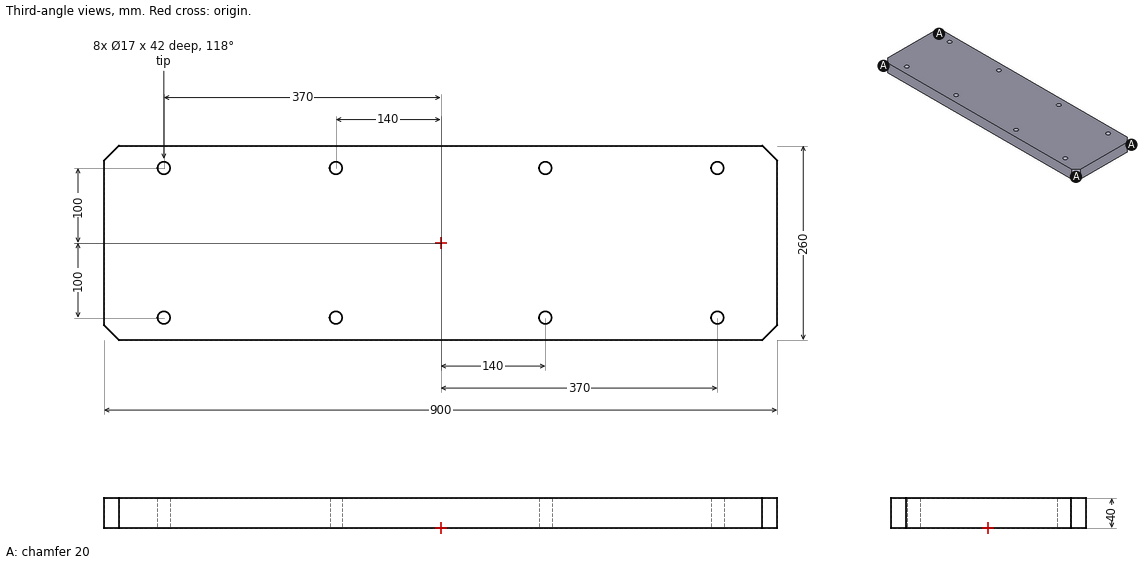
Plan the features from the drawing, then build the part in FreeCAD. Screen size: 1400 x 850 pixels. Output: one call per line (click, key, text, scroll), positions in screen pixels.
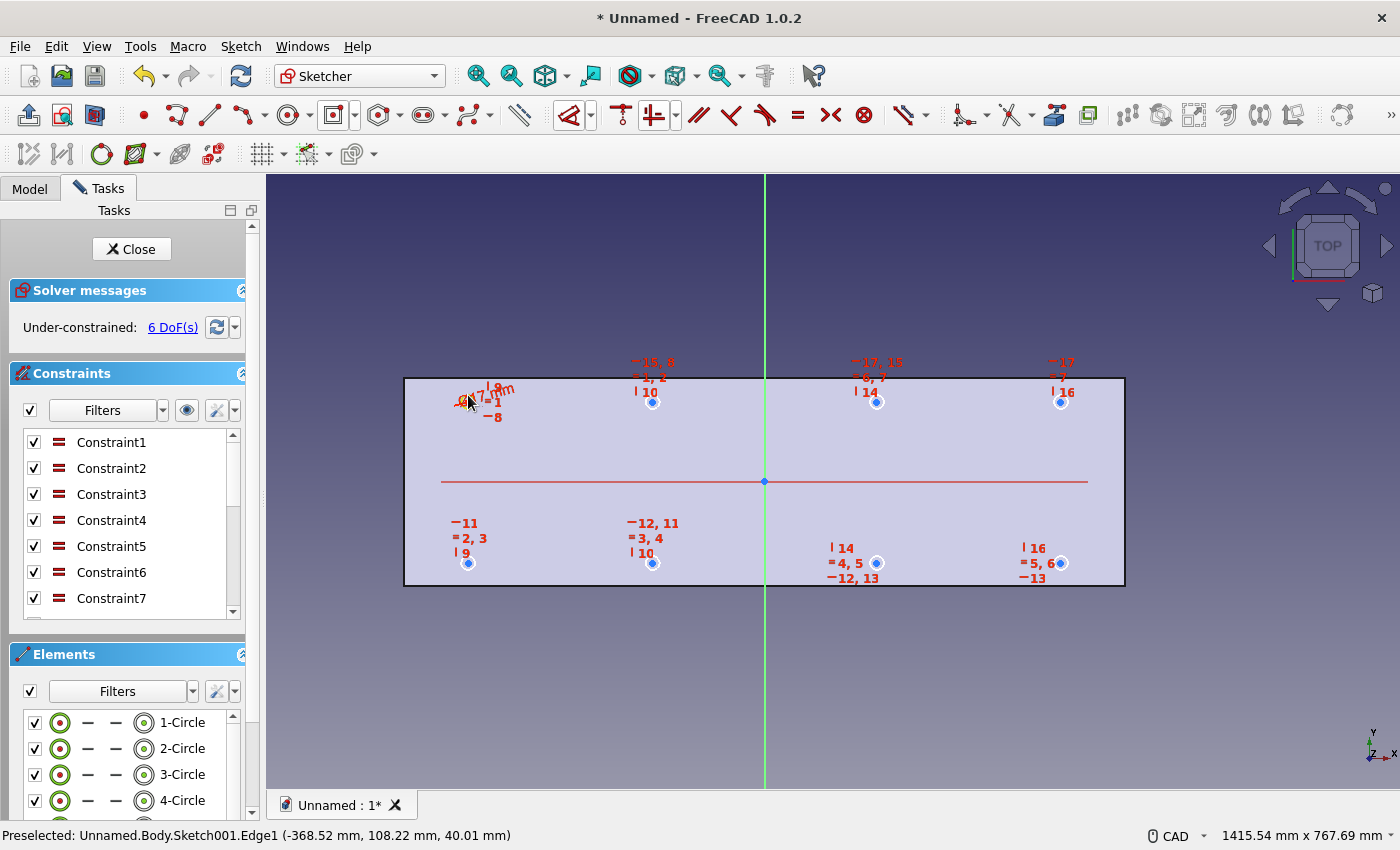
click(468, 402)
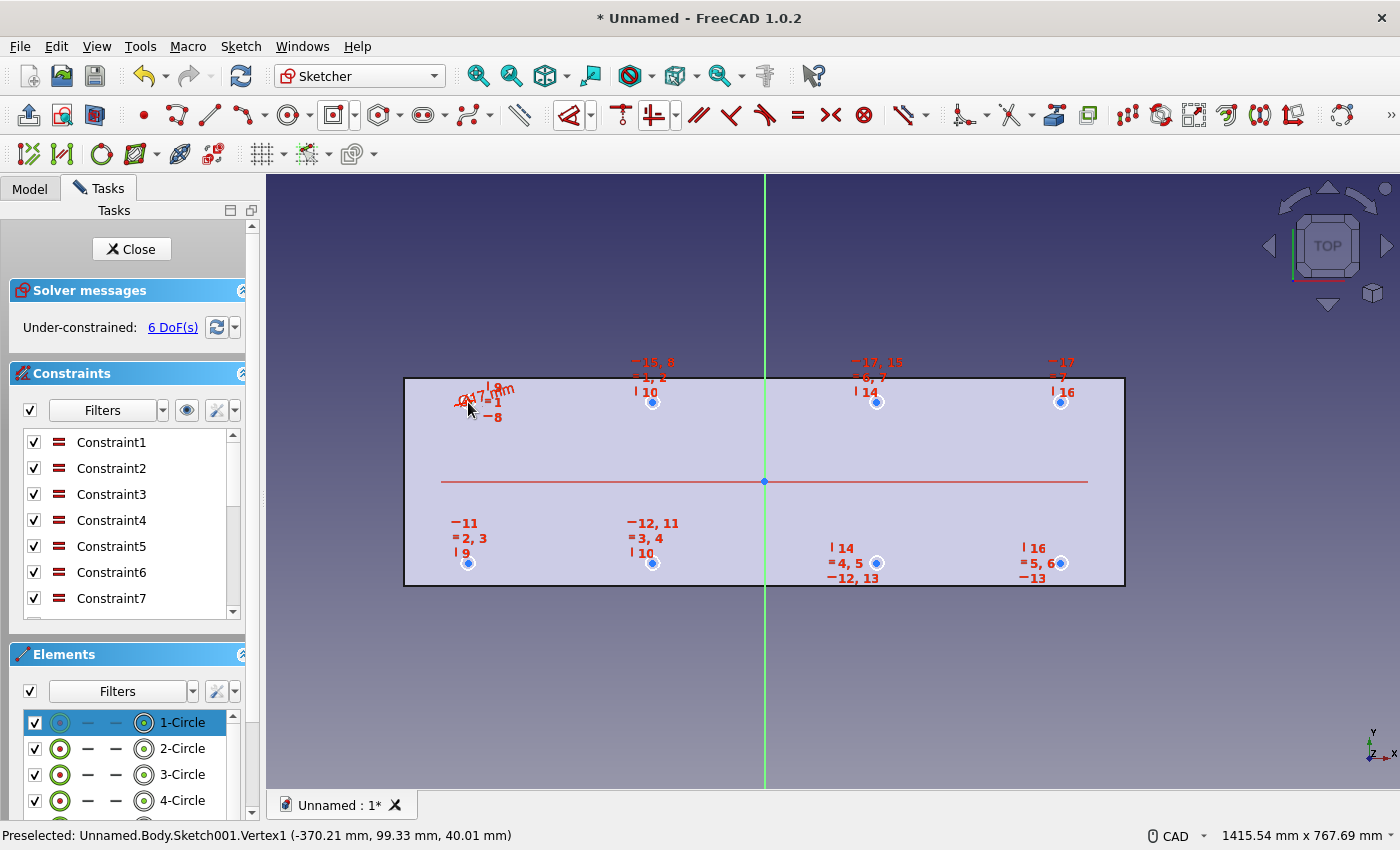
key(l)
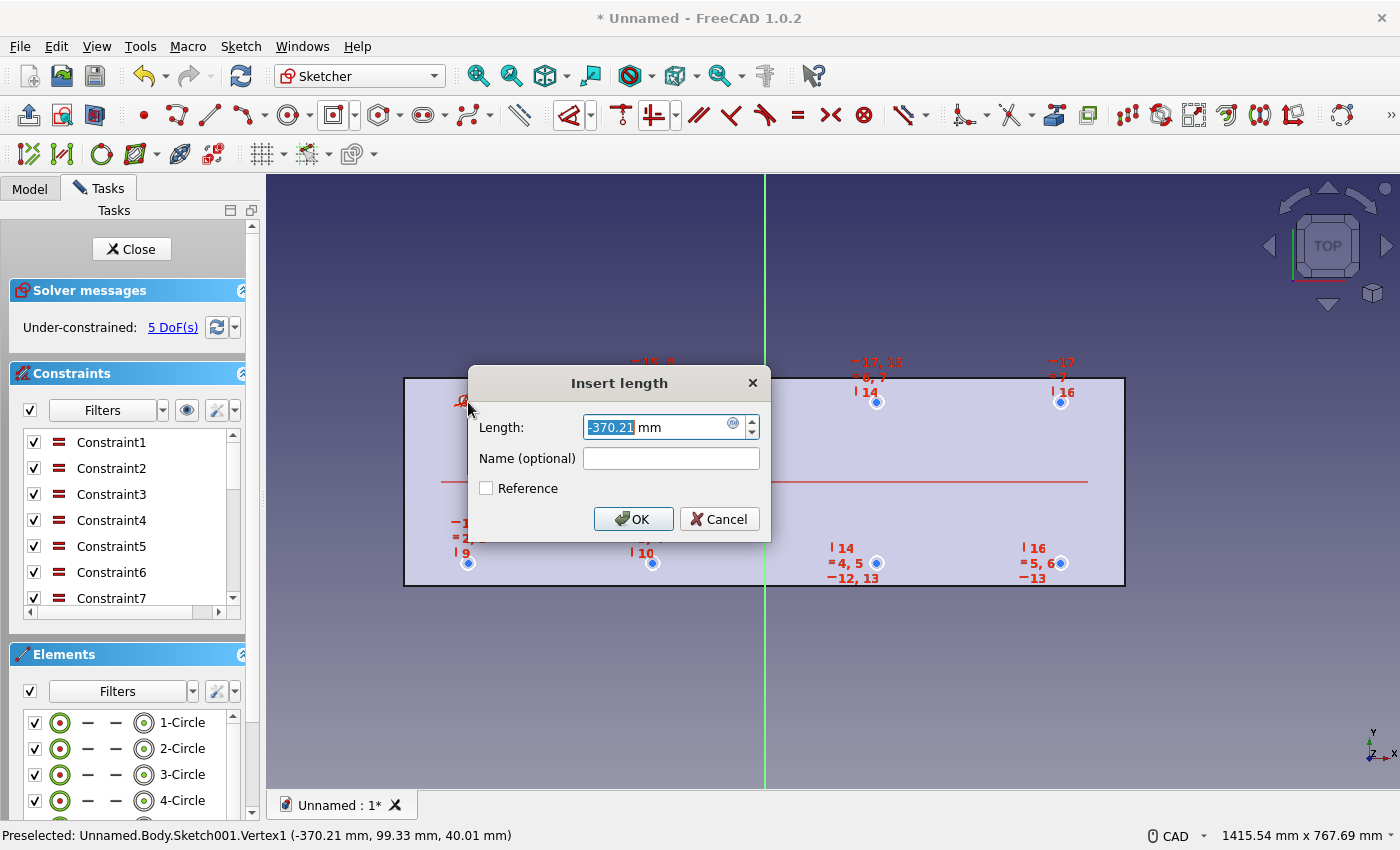
text(-370)
key(Return)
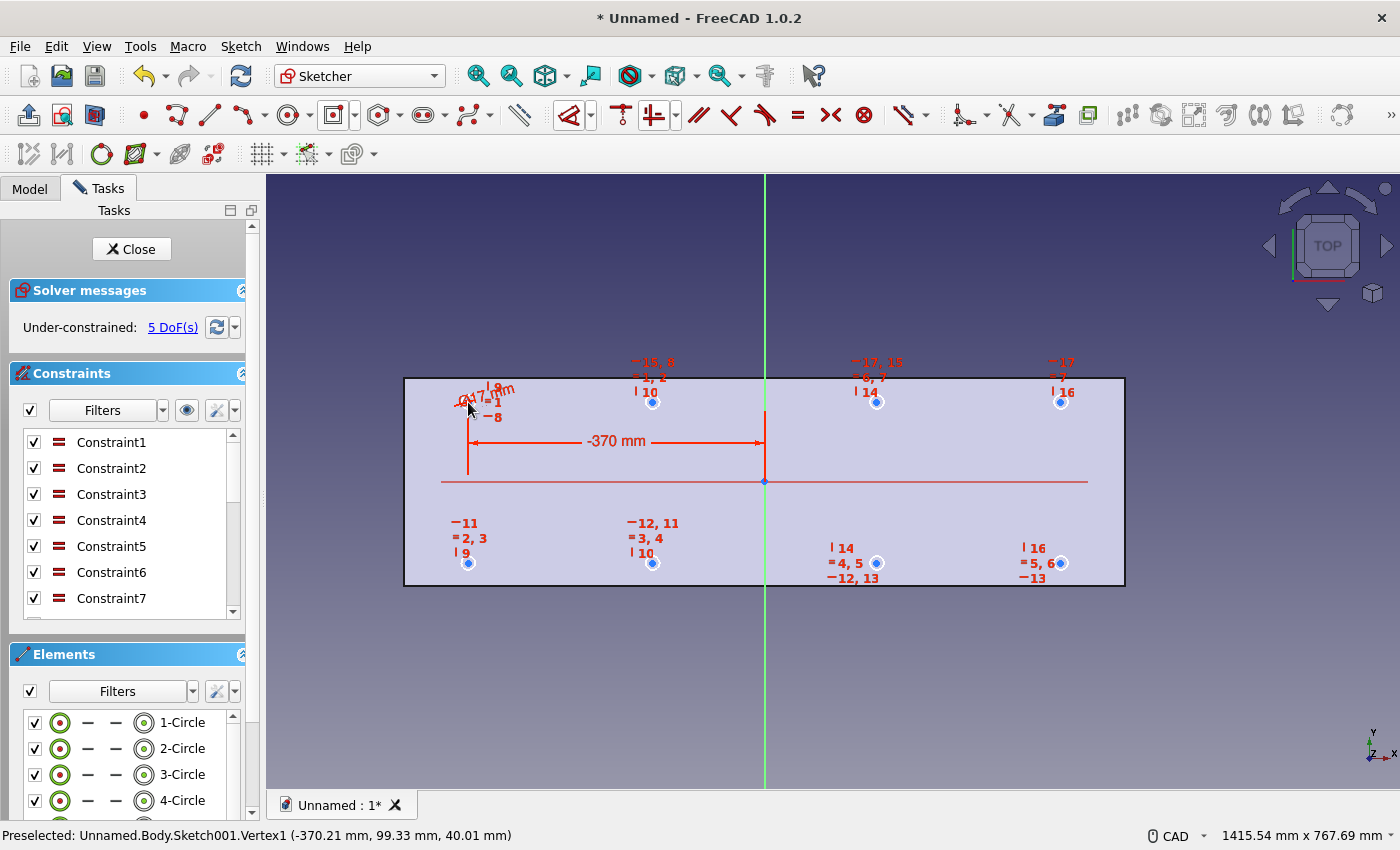
click(468, 402)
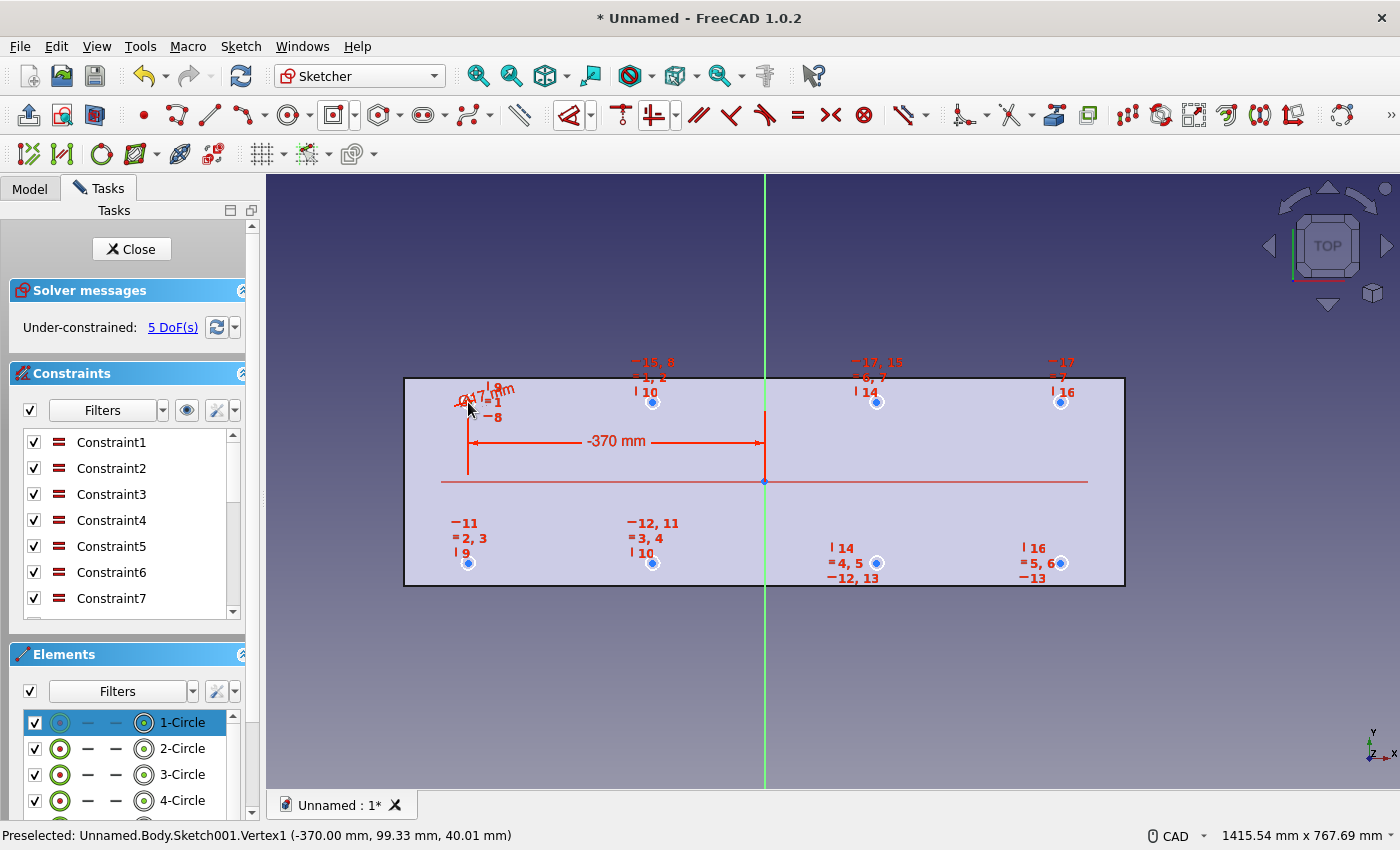
click(590, 116)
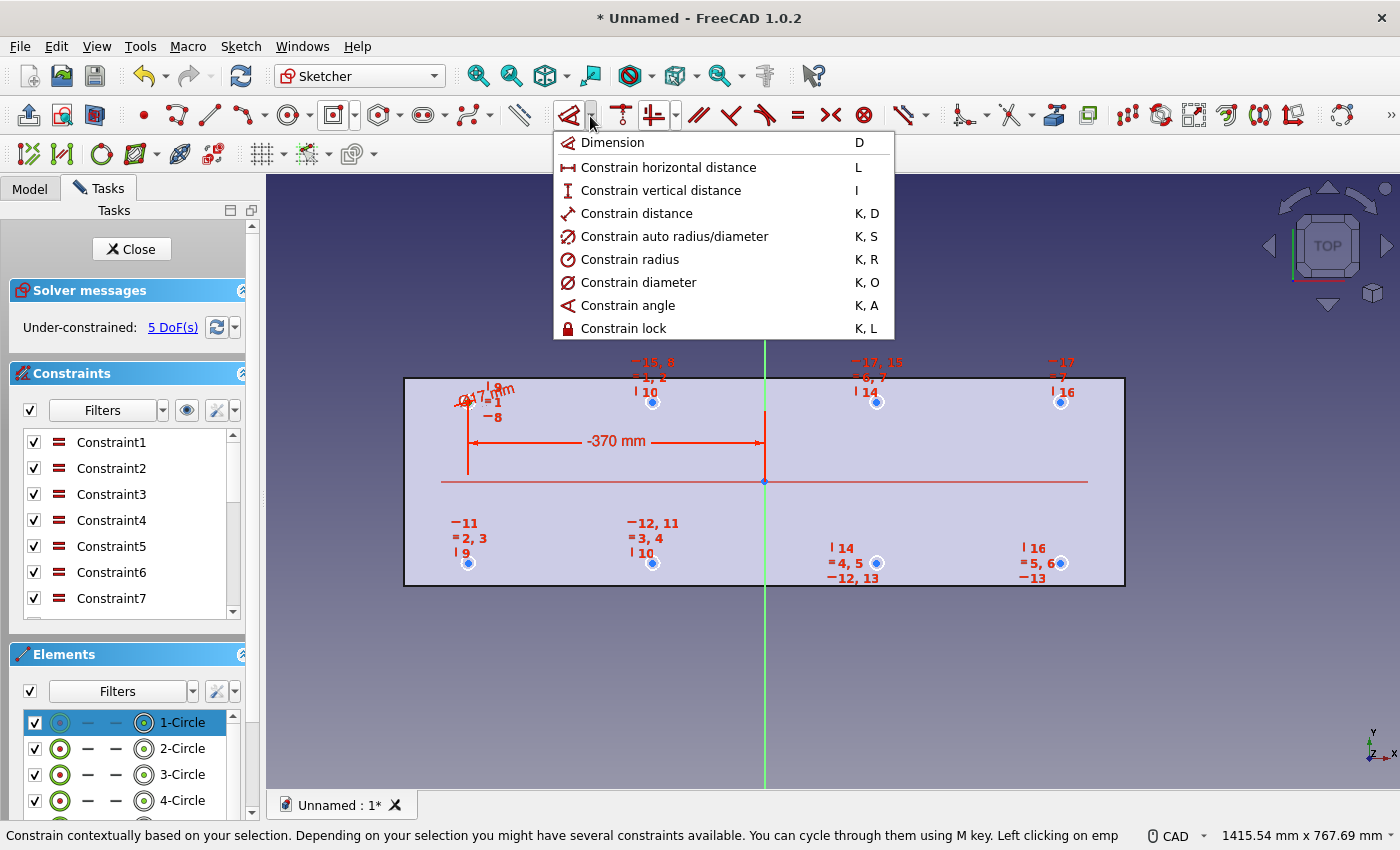
click(724, 190)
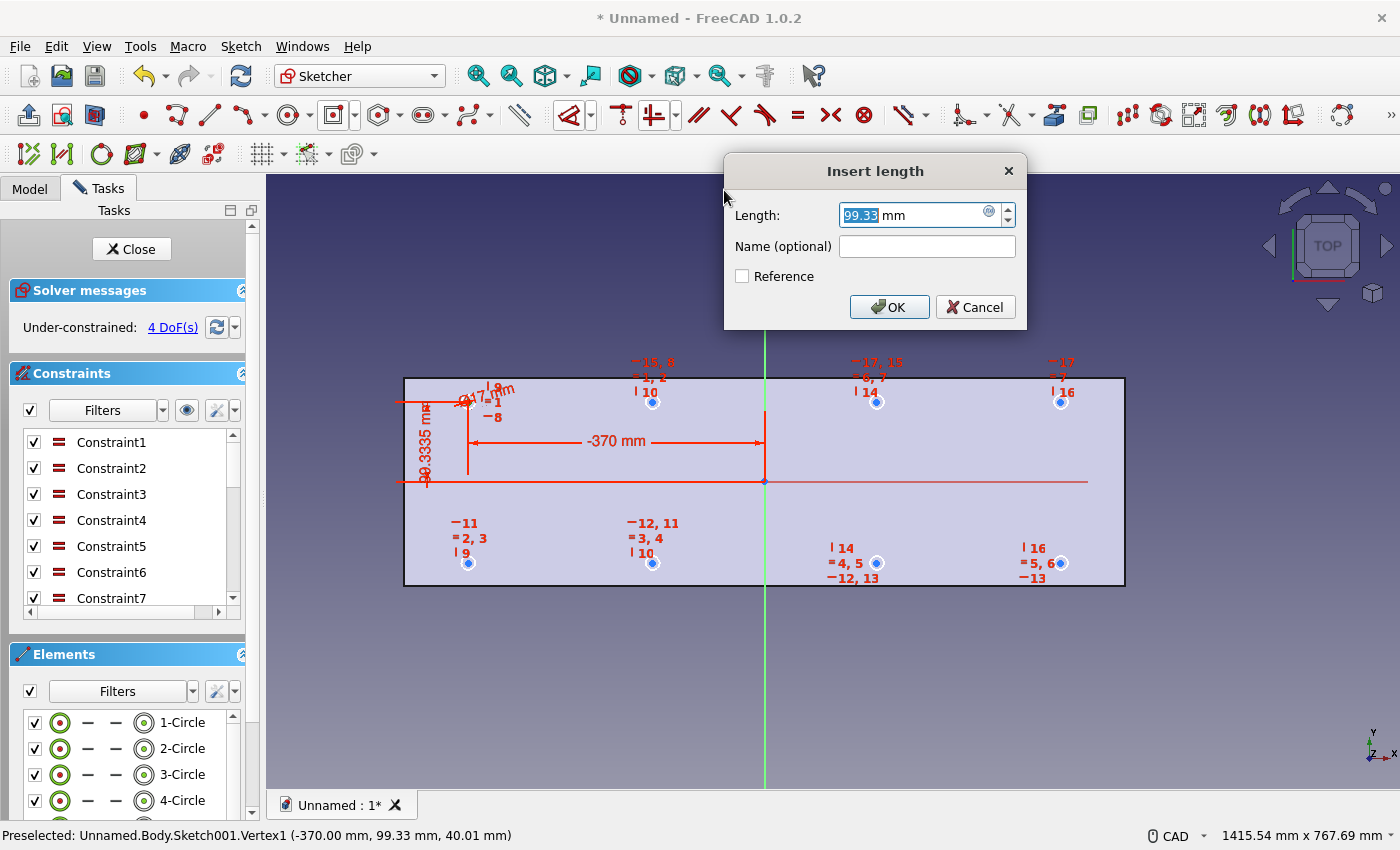
text(100)
key(Return)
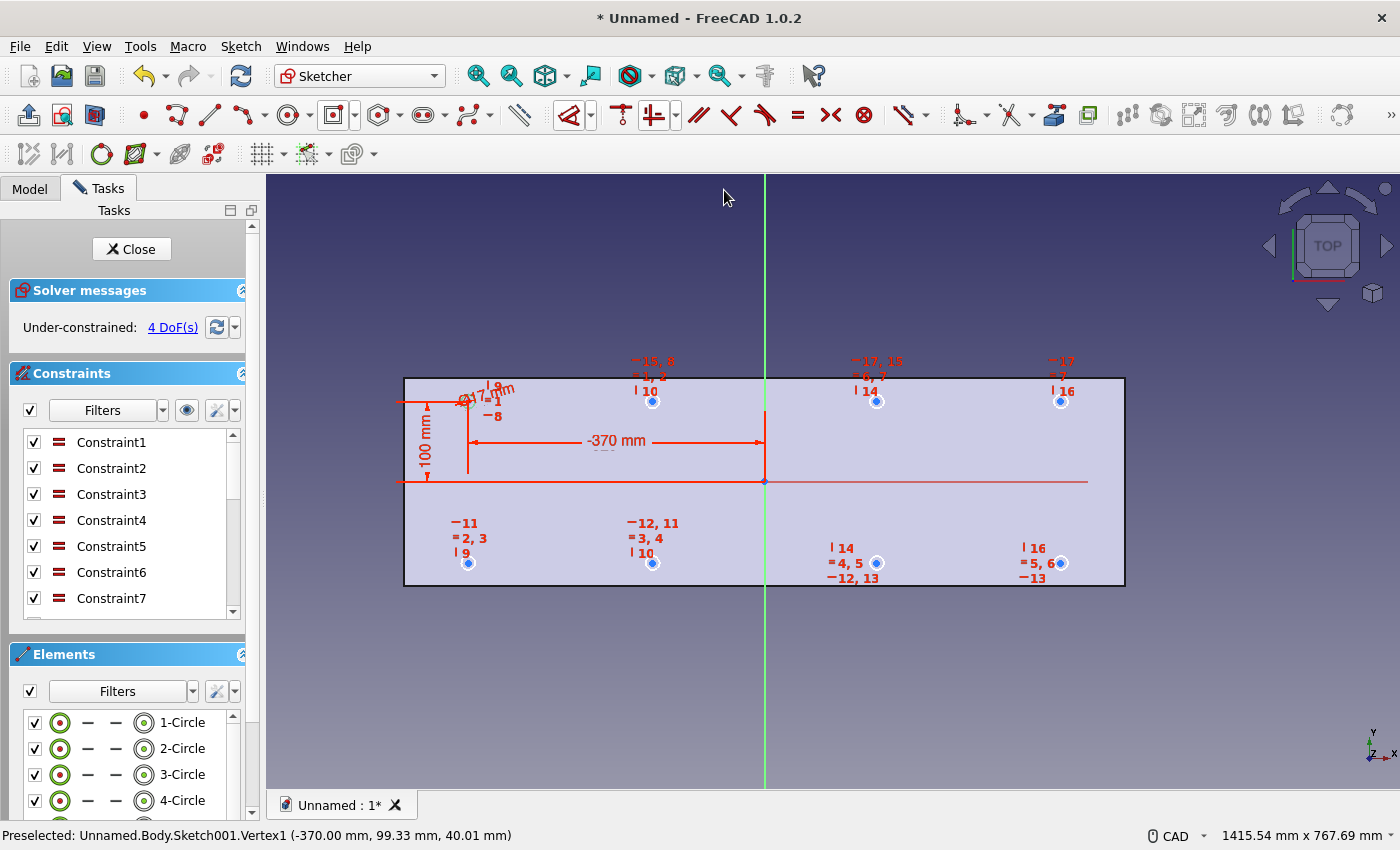
click(653, 402)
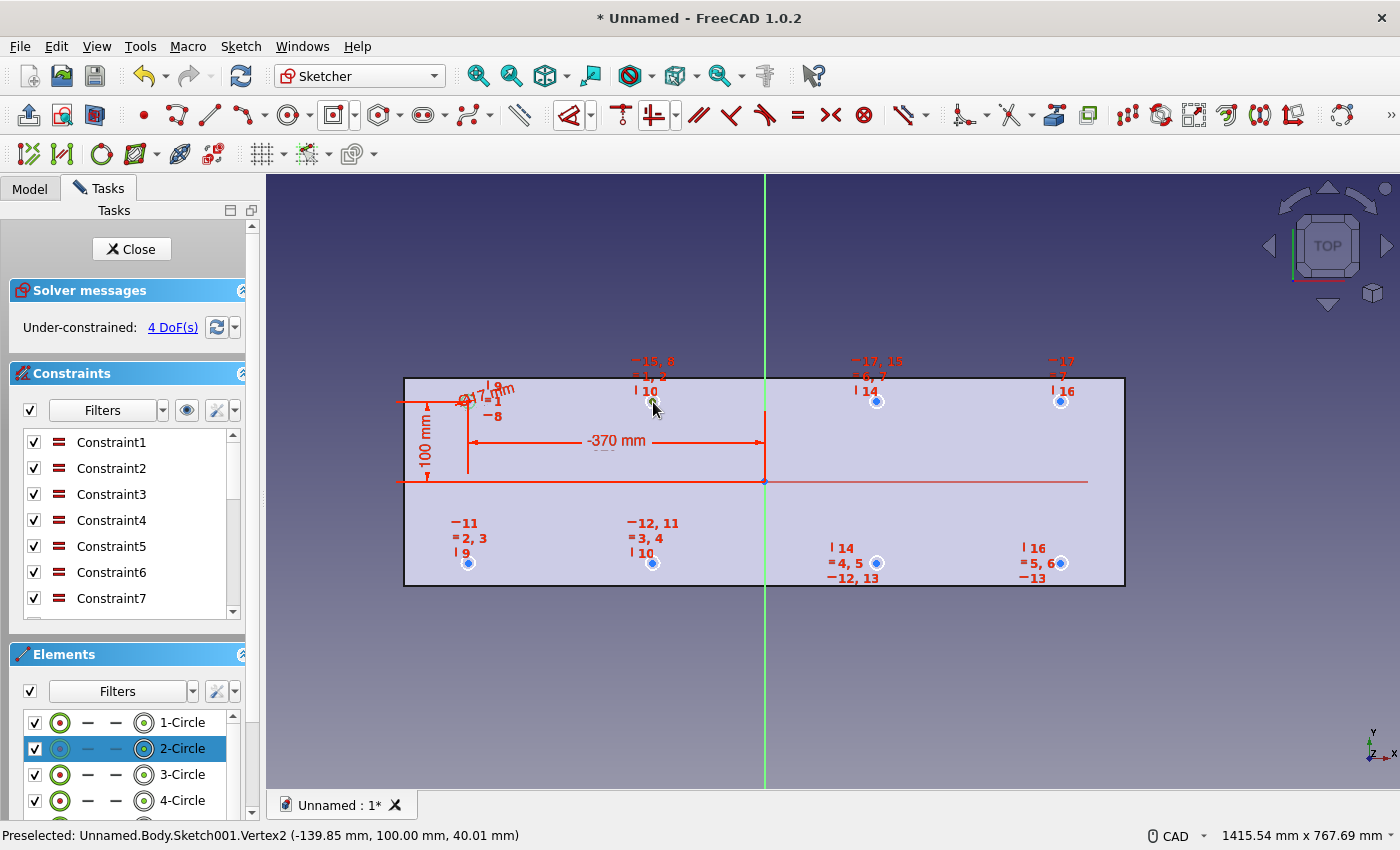
click(590, 116)